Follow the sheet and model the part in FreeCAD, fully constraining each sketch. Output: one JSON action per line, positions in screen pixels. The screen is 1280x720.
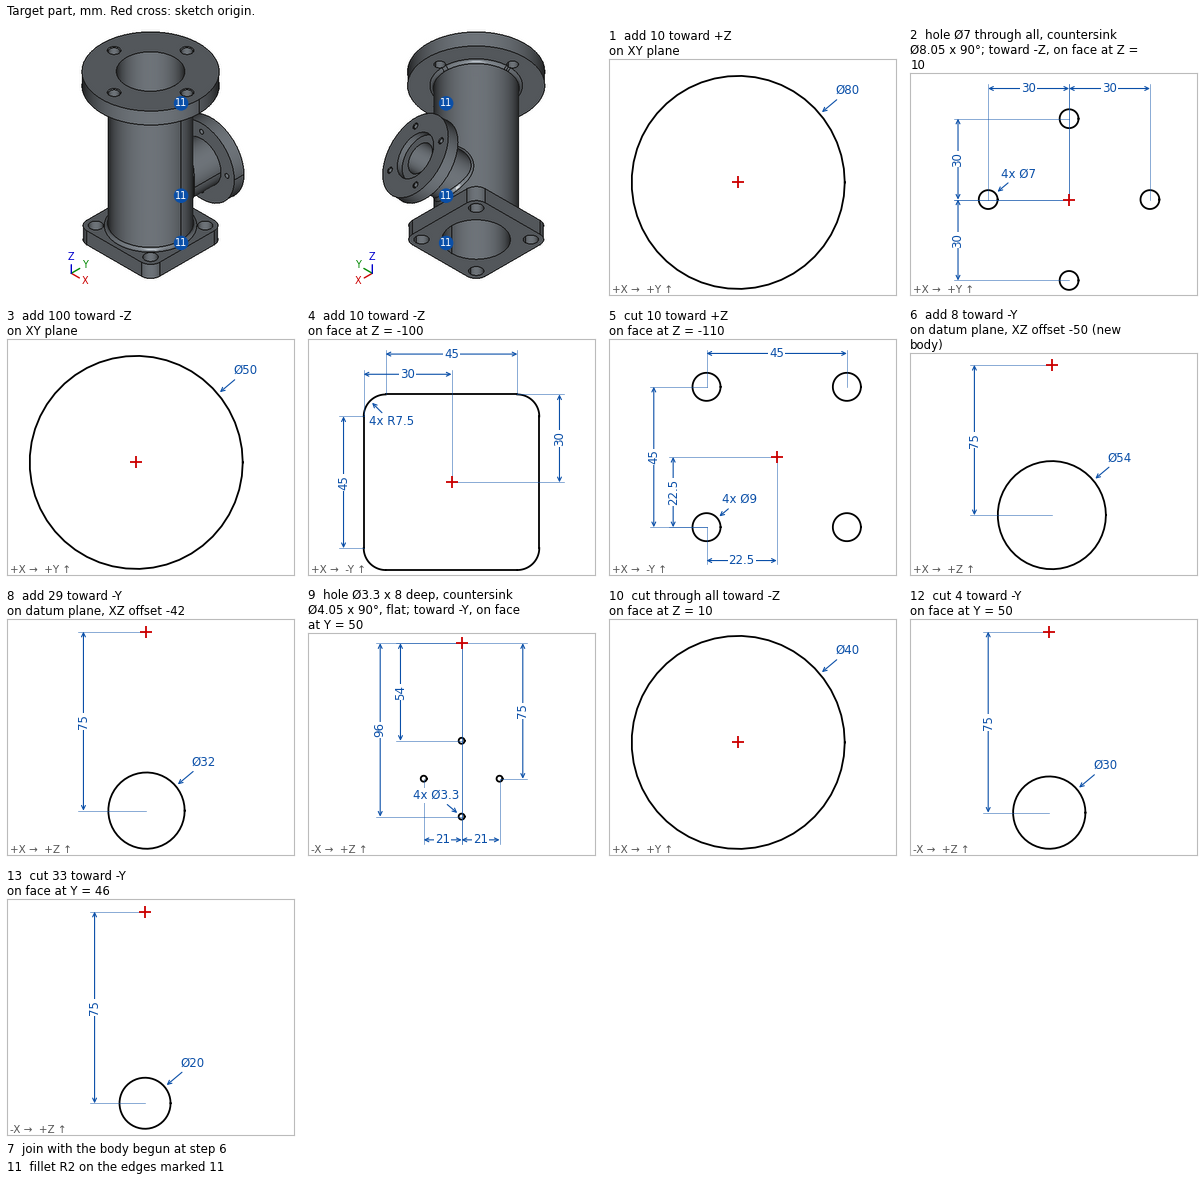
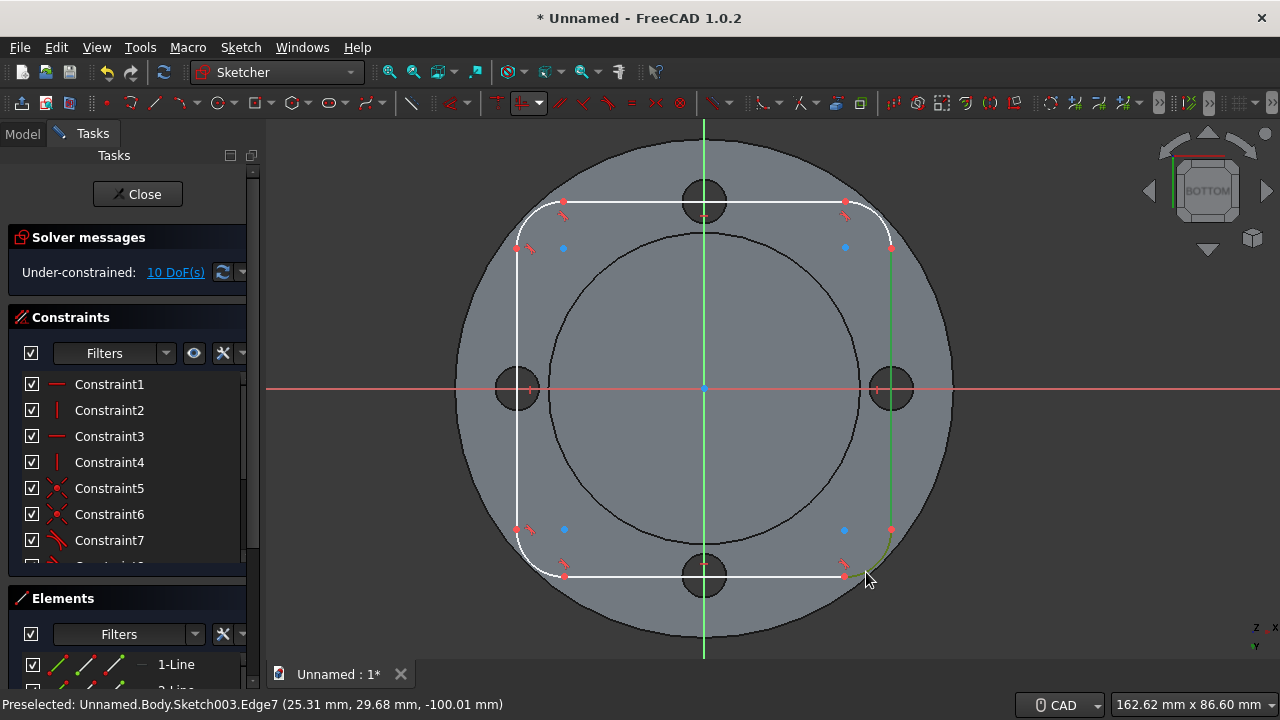
{"action": "left_click", "coordinate": [608, 104]}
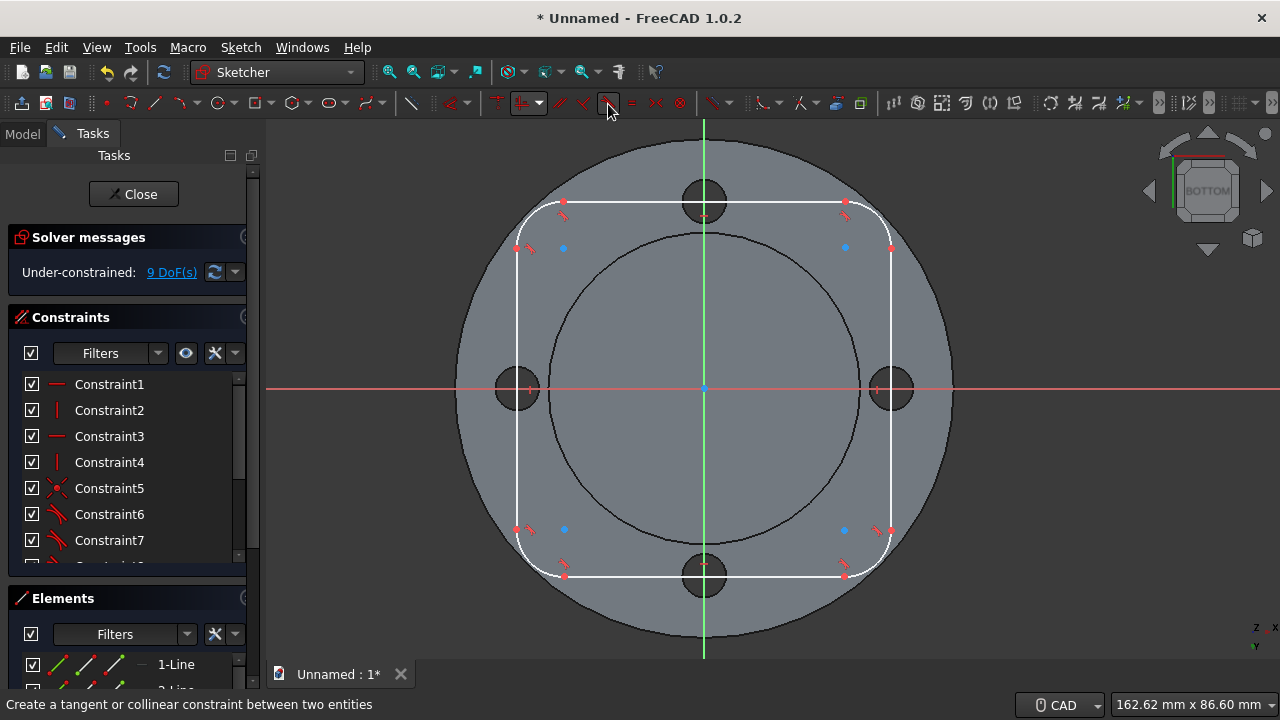
{"action": "left_click", "coordinate": [891, 446]}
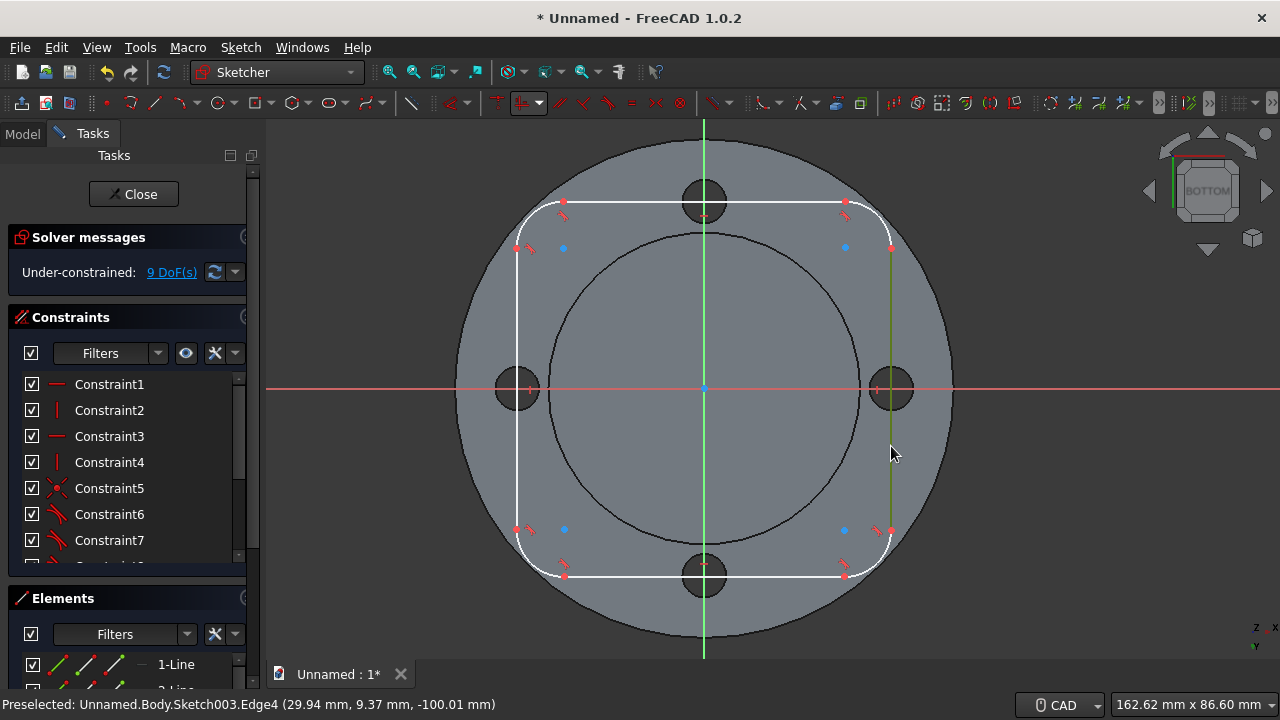
{"action": "left_click", "coordinate": [886, 228]}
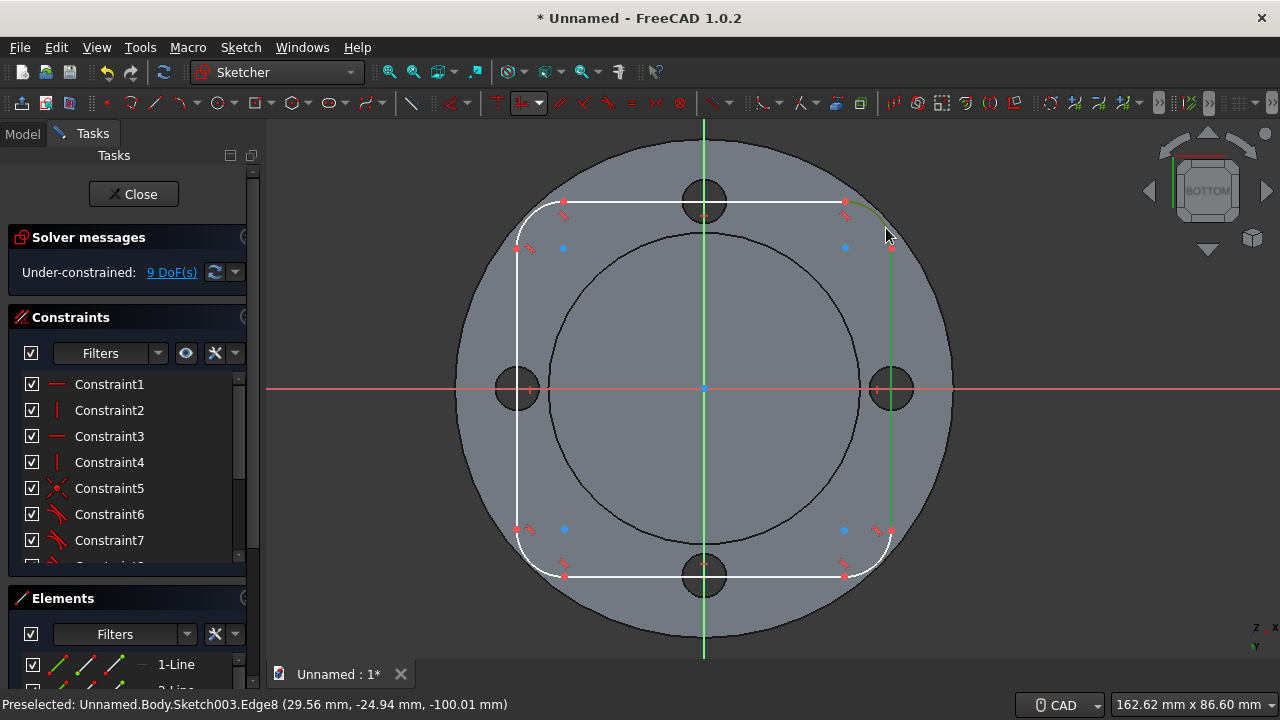
{"action": "left_click", "coordinate": [608, 104]}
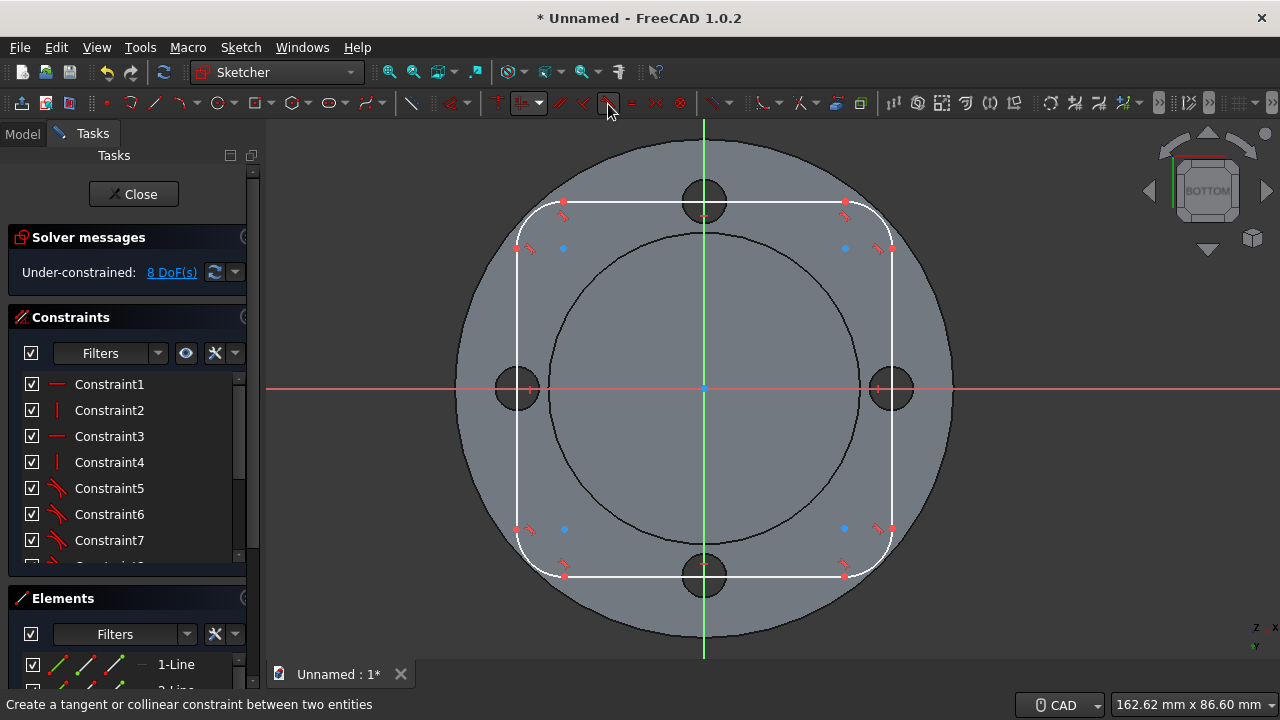
{"action": "left_click", "coordinate": [543, 207]}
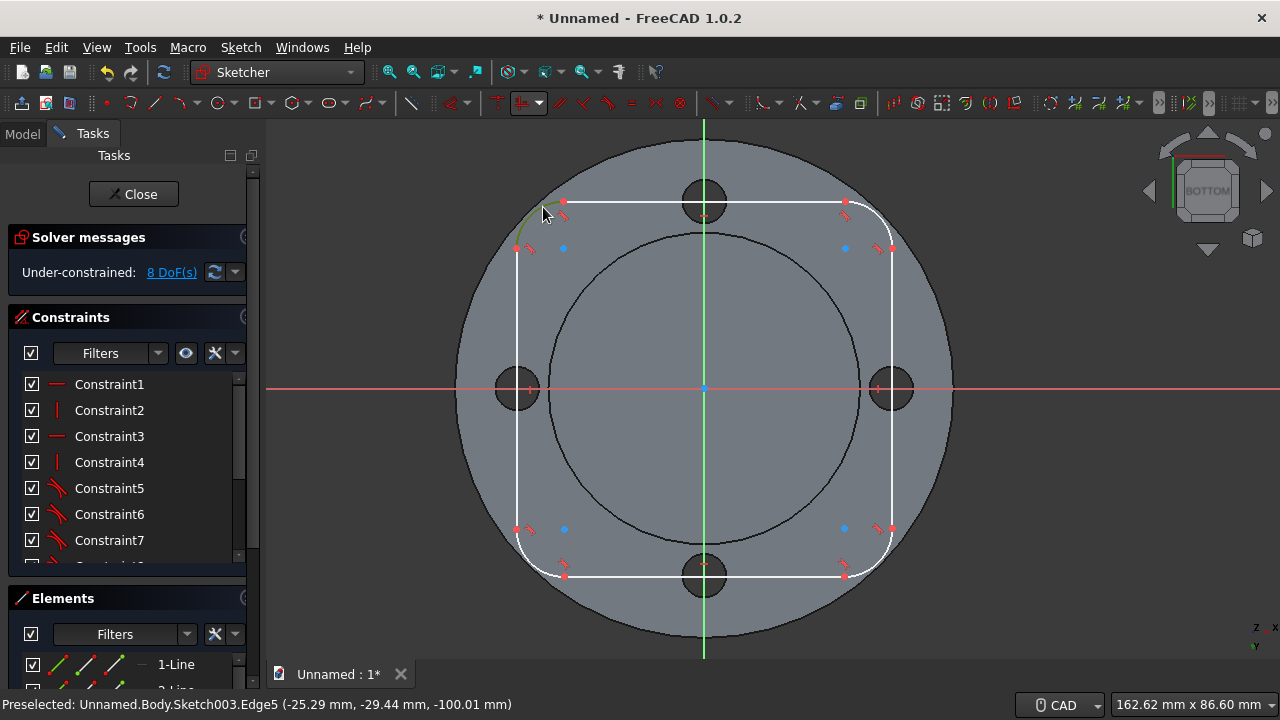
{"action": "left_click", "coordinate": [522, 551]}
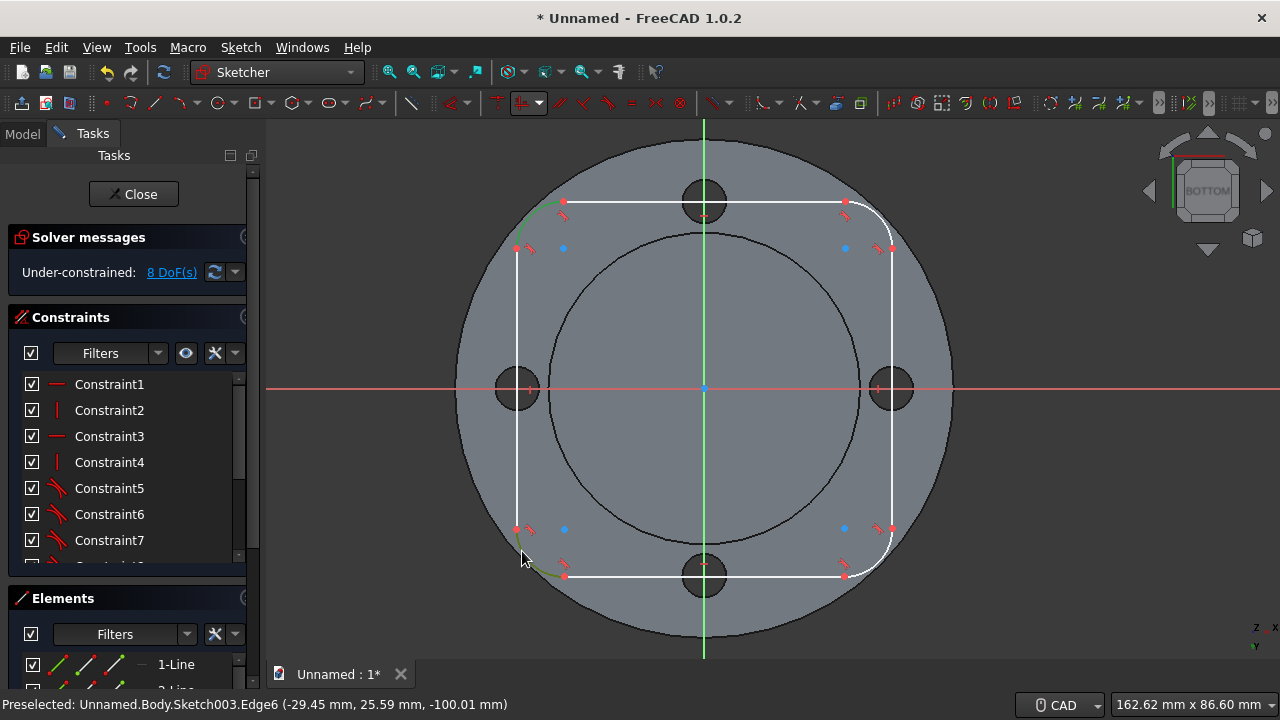
{"action": "left_click", "coordinate": [866, 572]}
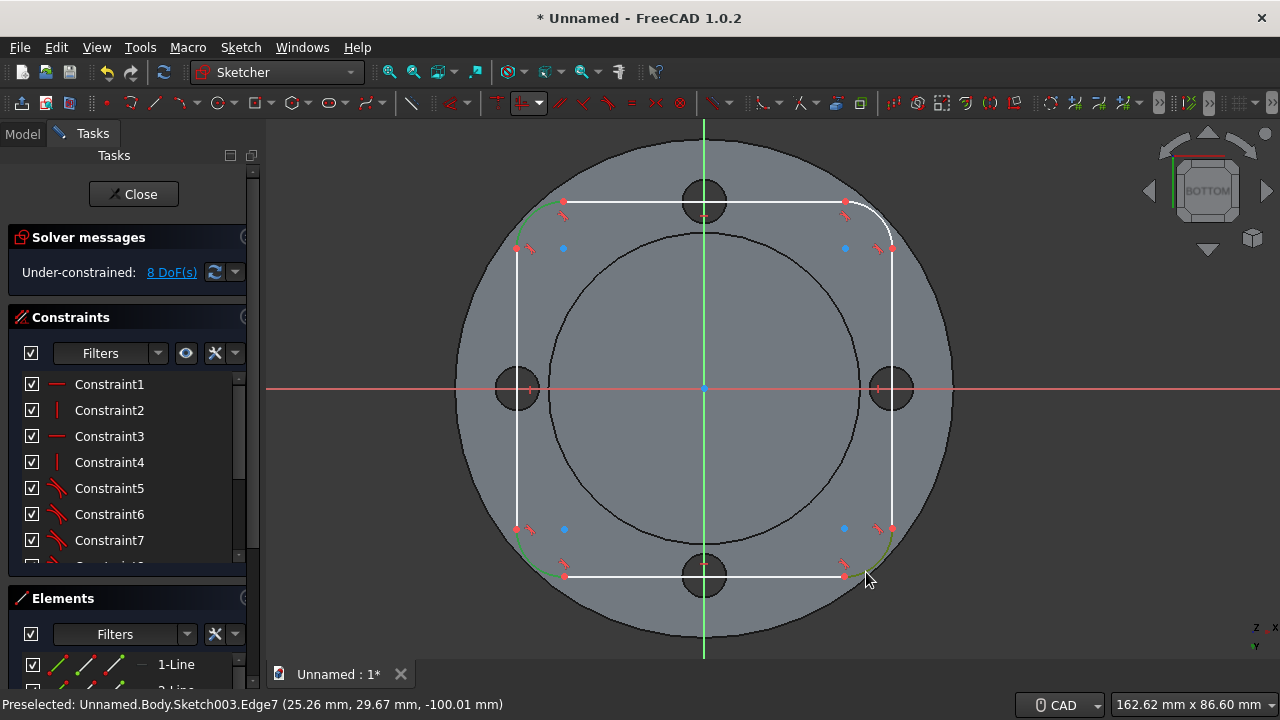
{"action": "left_click", "coordinate": [887, 228]}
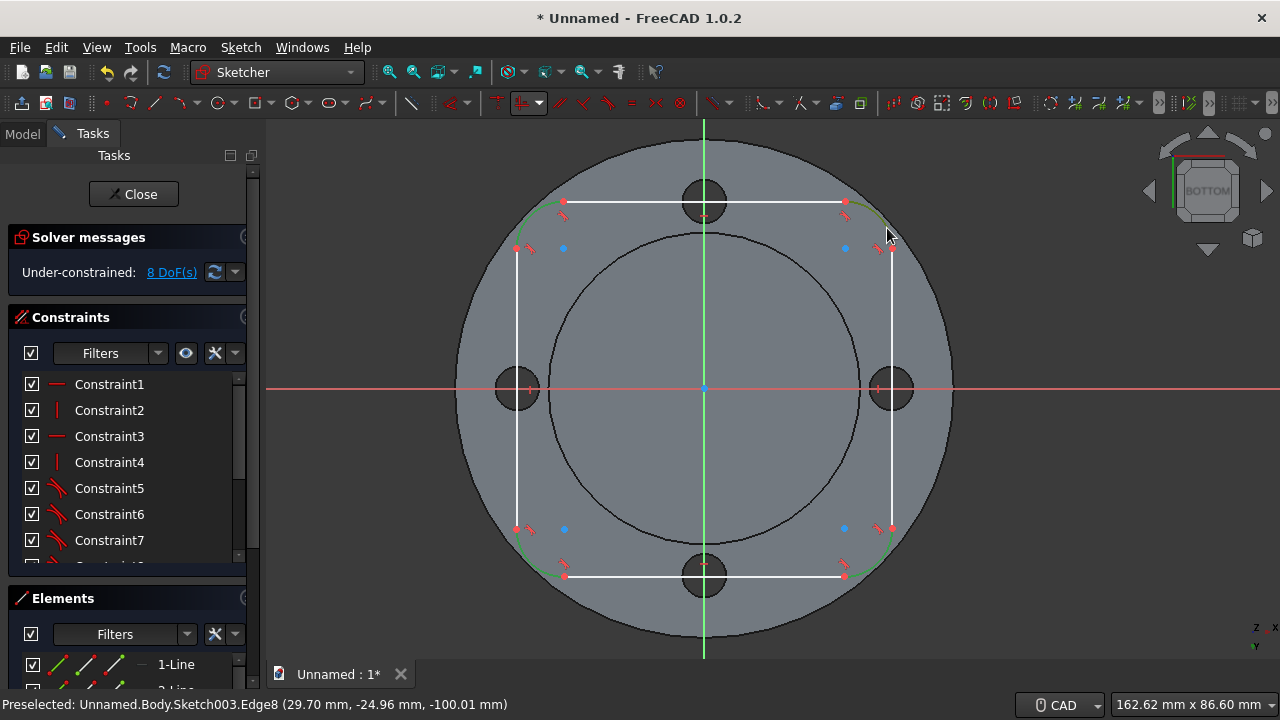
{"action": "left_click", "coordinate": [632, 104]}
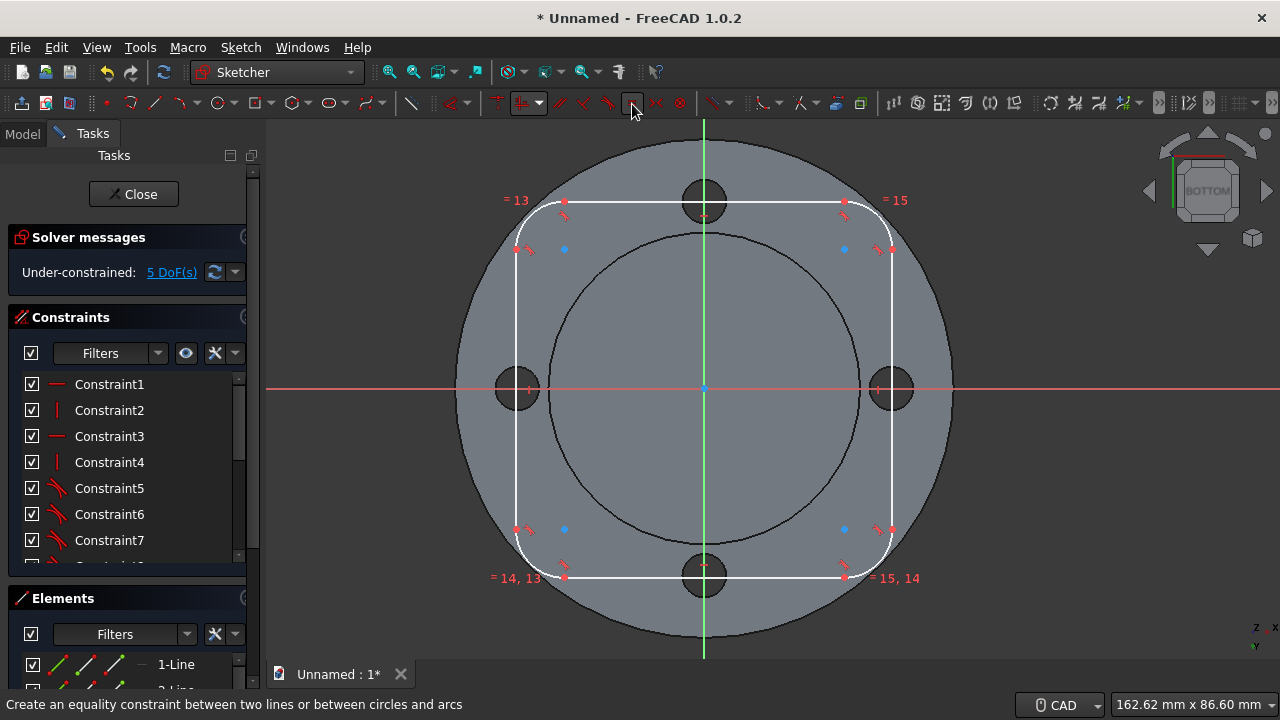
{"action": "left_click", "coordinate": [450, 104]}